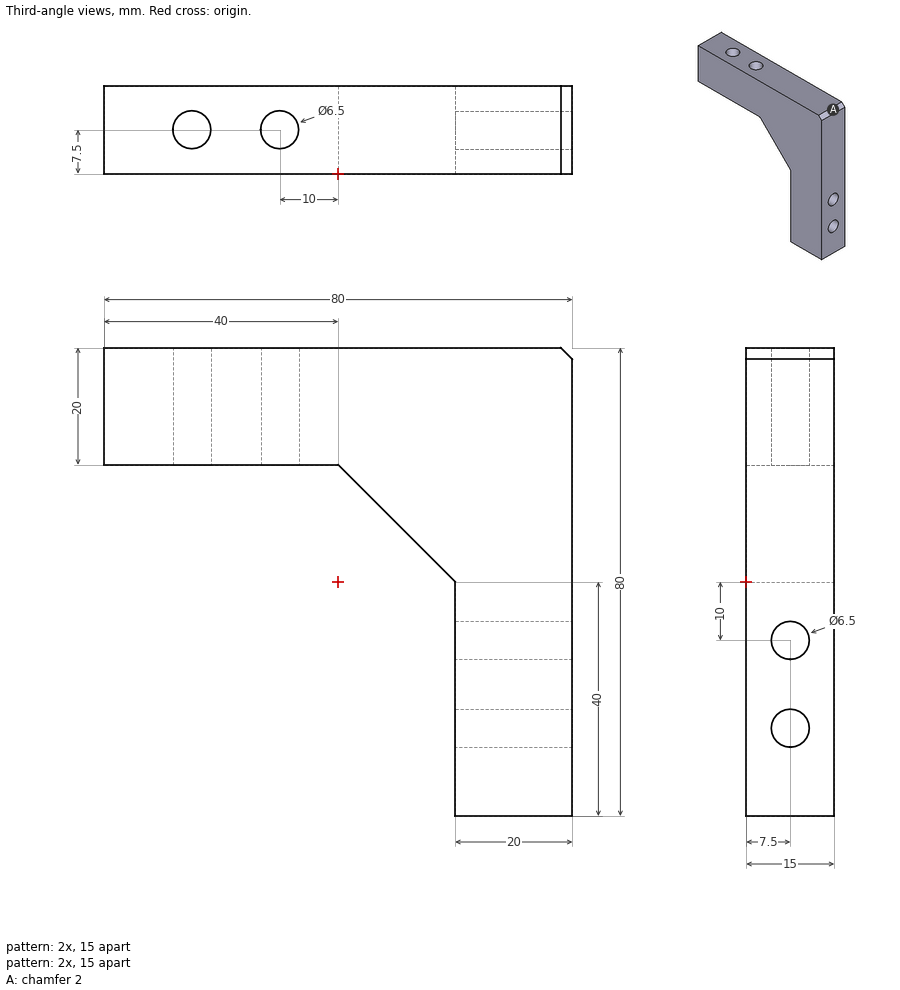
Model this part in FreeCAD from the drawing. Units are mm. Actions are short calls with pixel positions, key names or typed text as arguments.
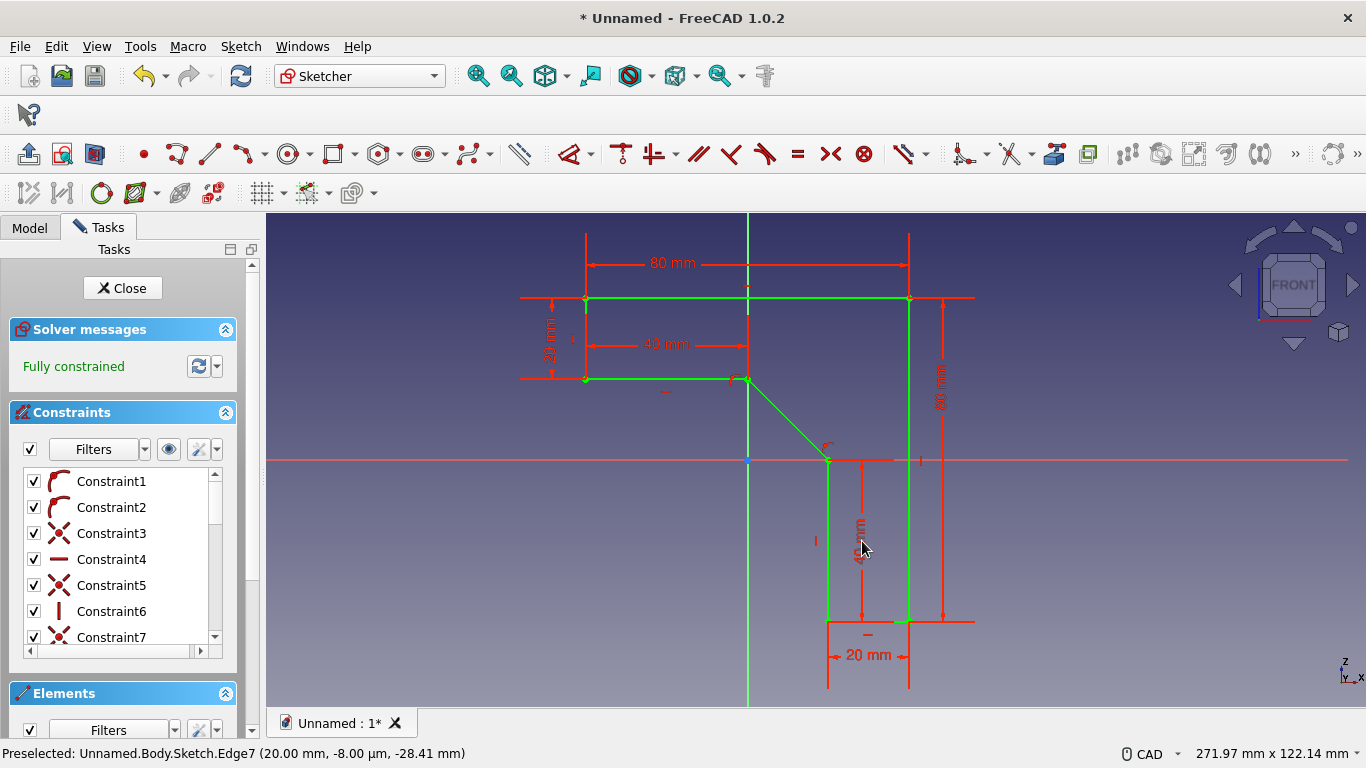
click(123, 288)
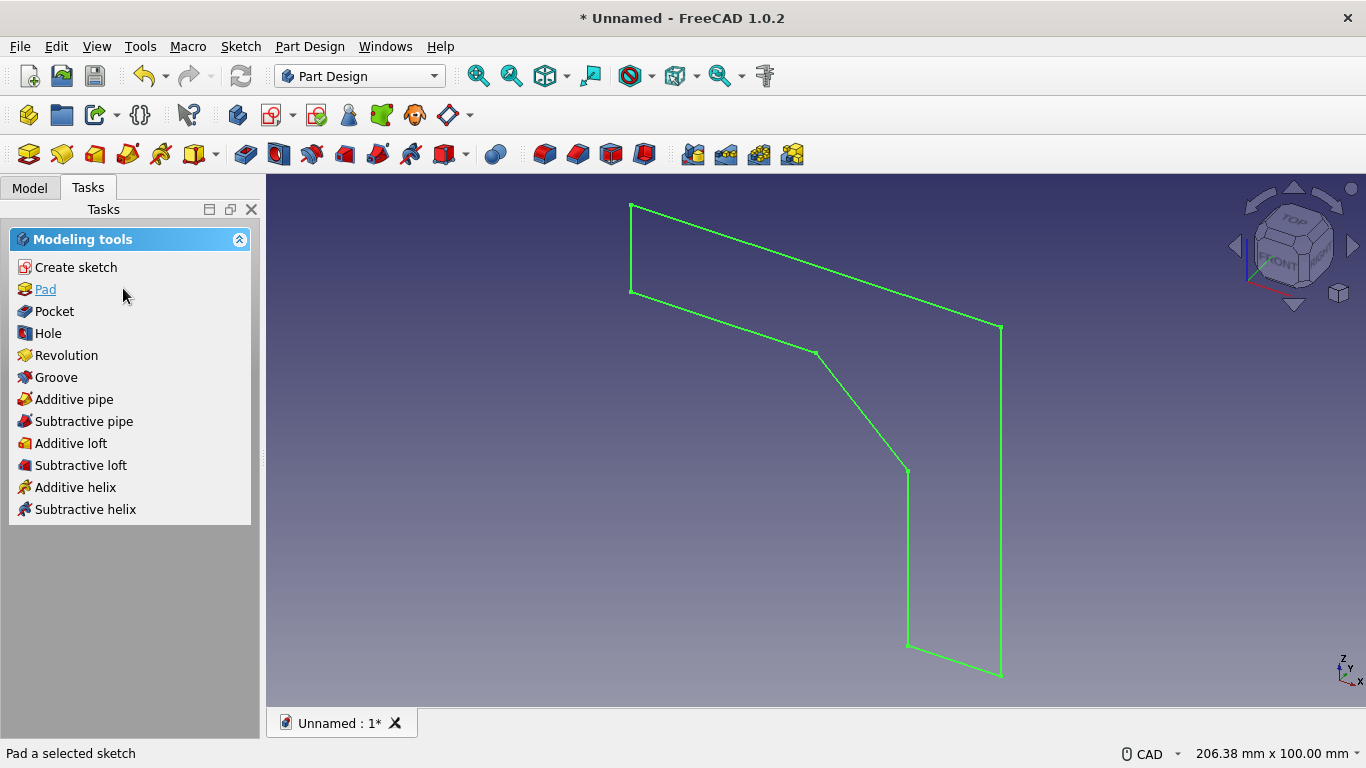
click(29, 154)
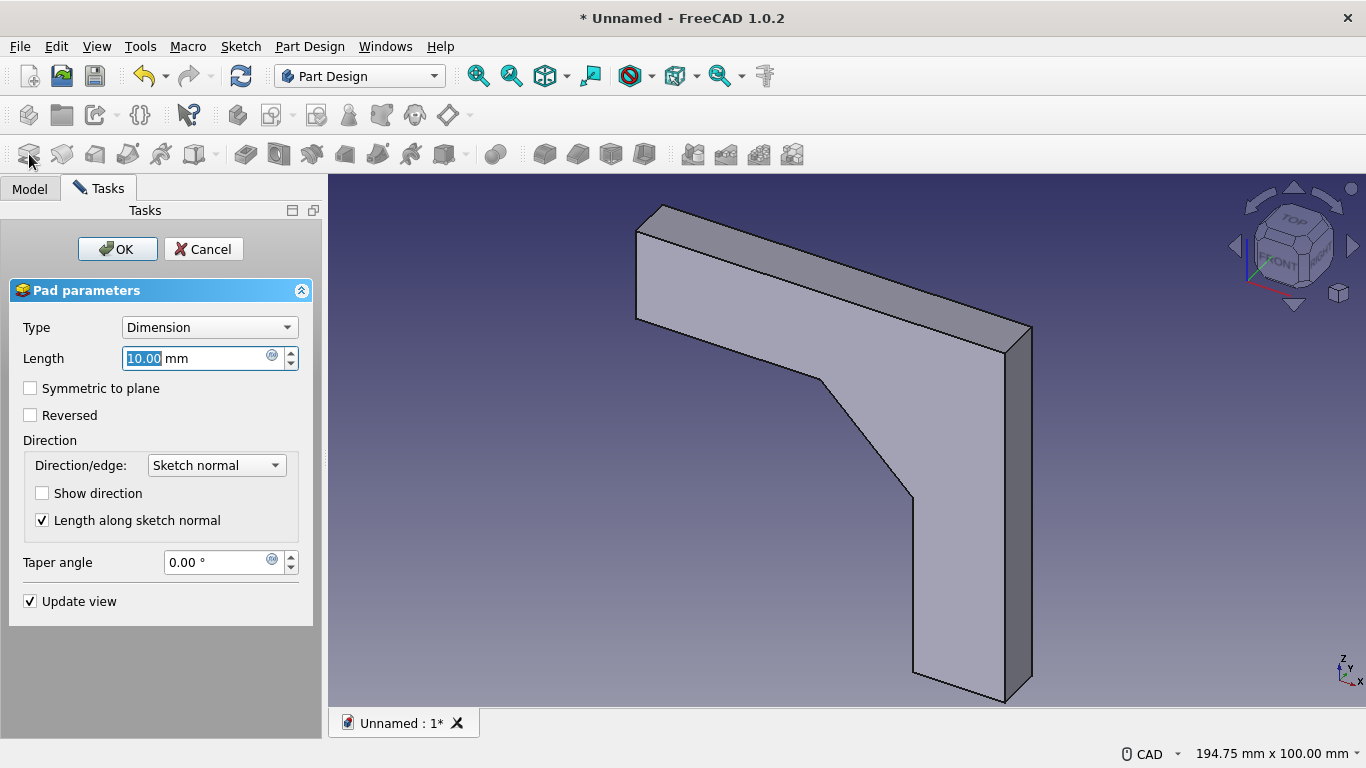
text(15)
key(Tab)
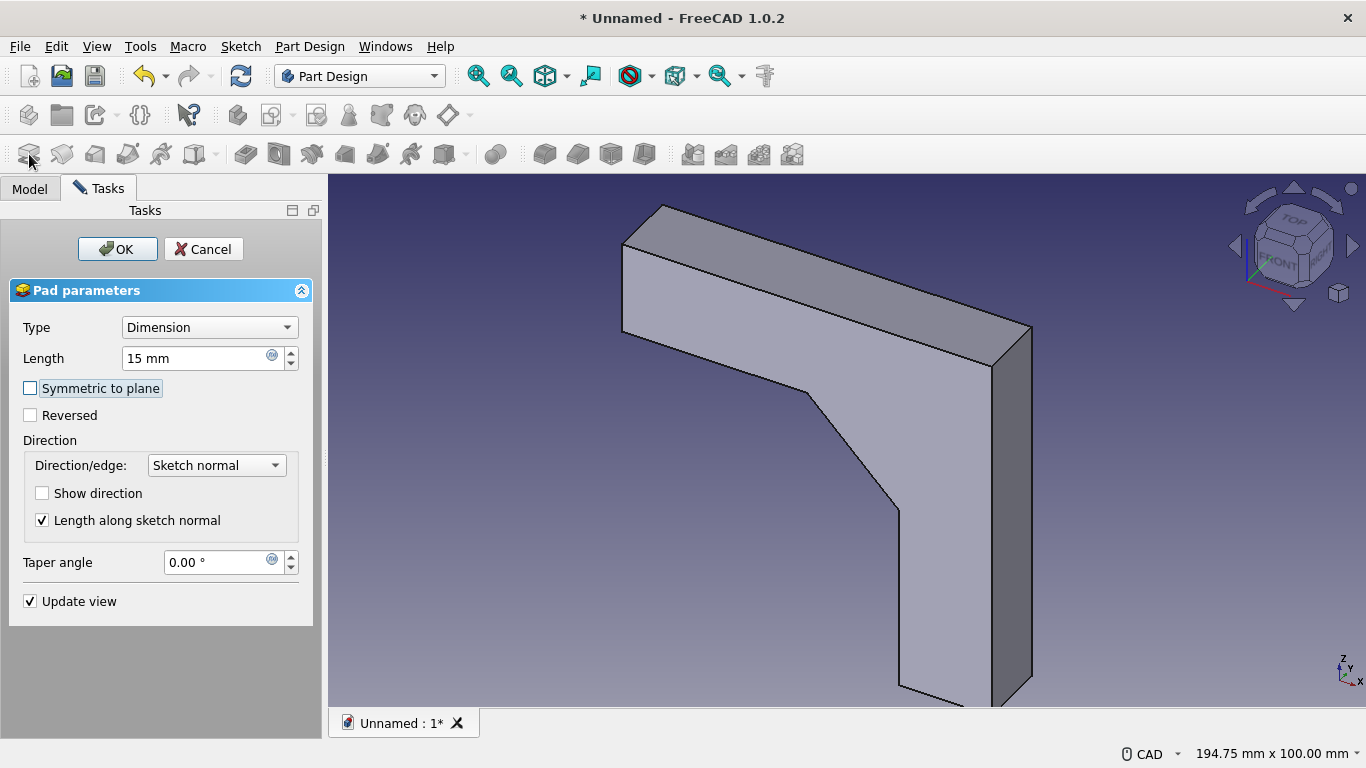
click(31, 415)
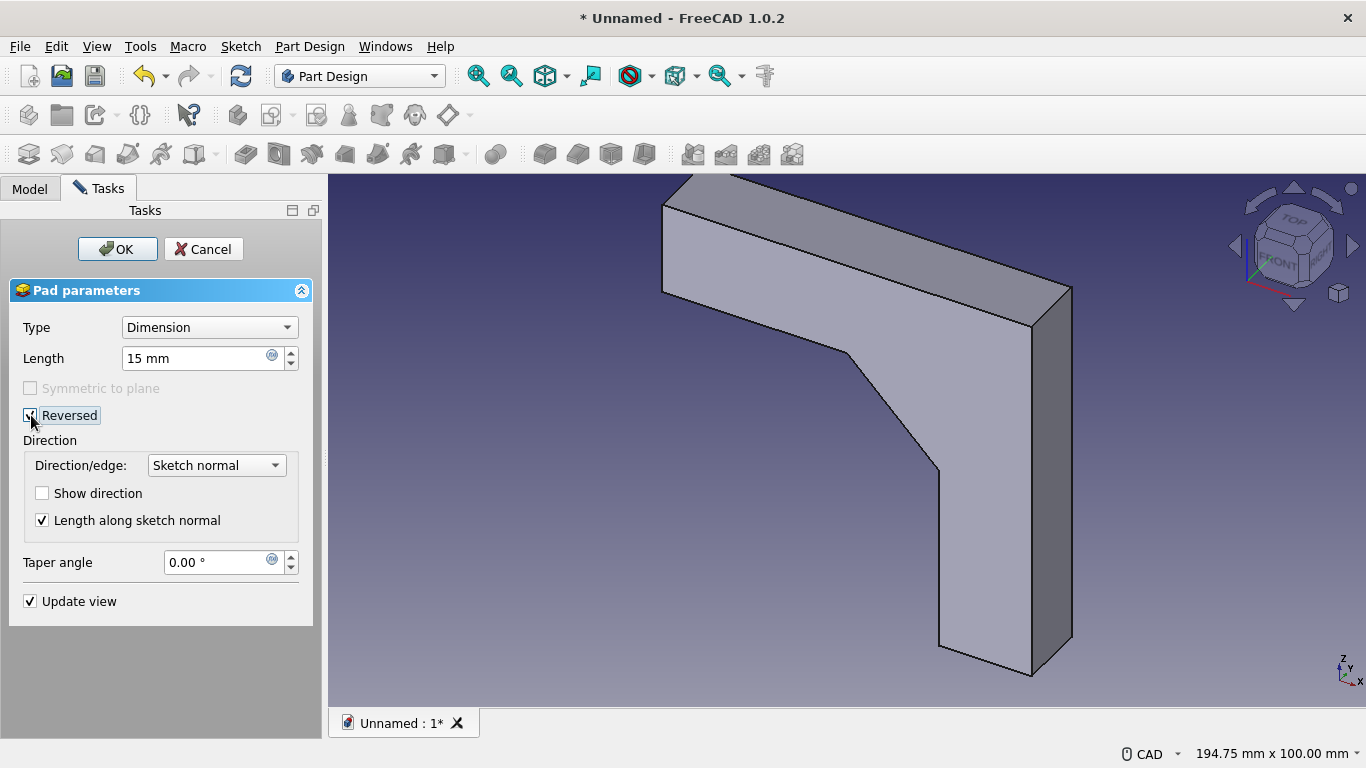
click(118, 249)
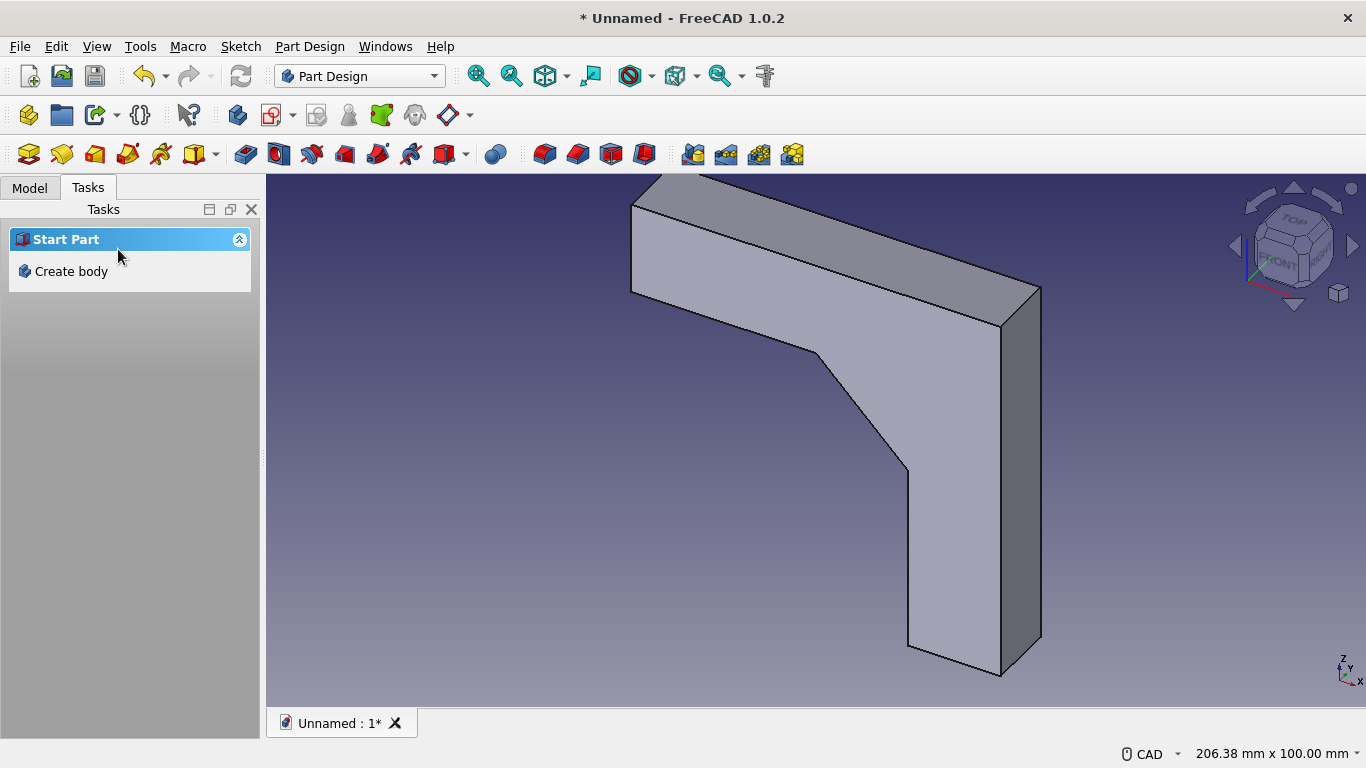
key(v)
key(f)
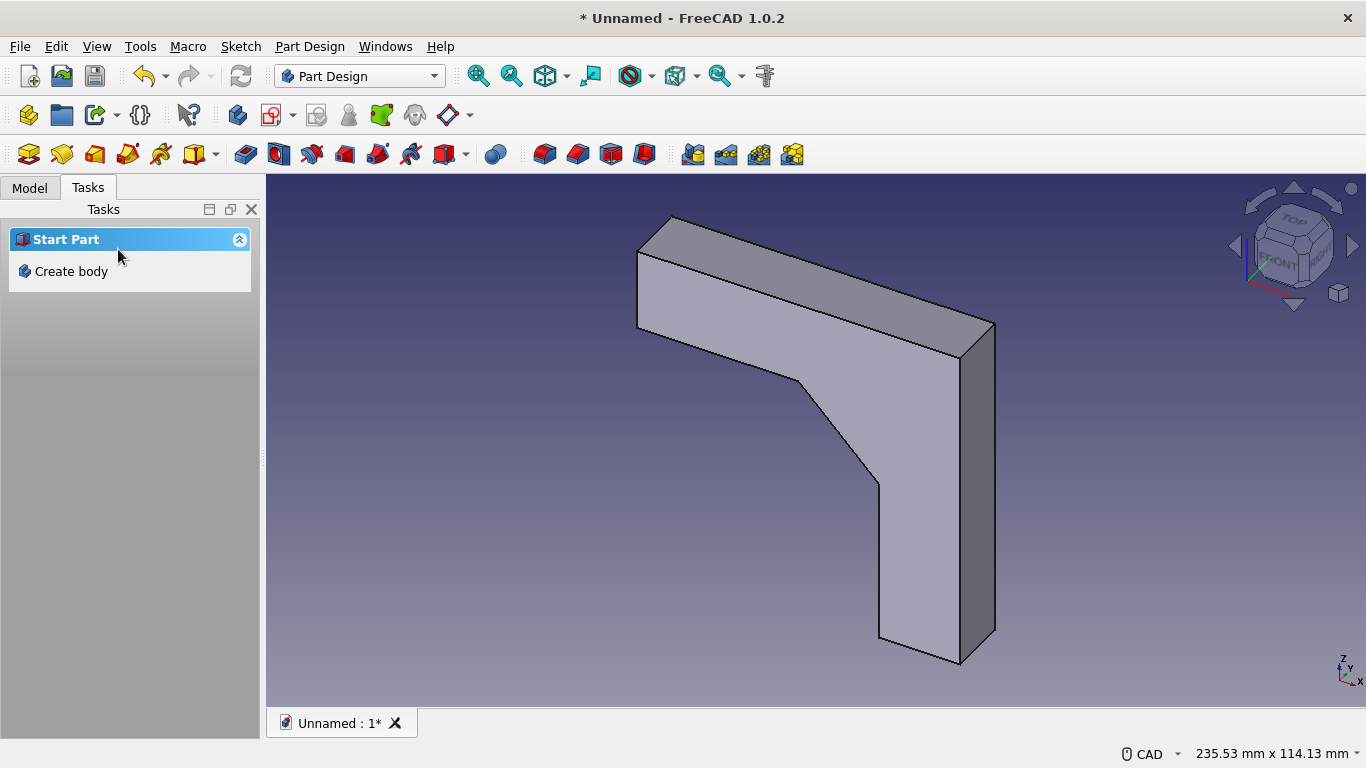
key(5)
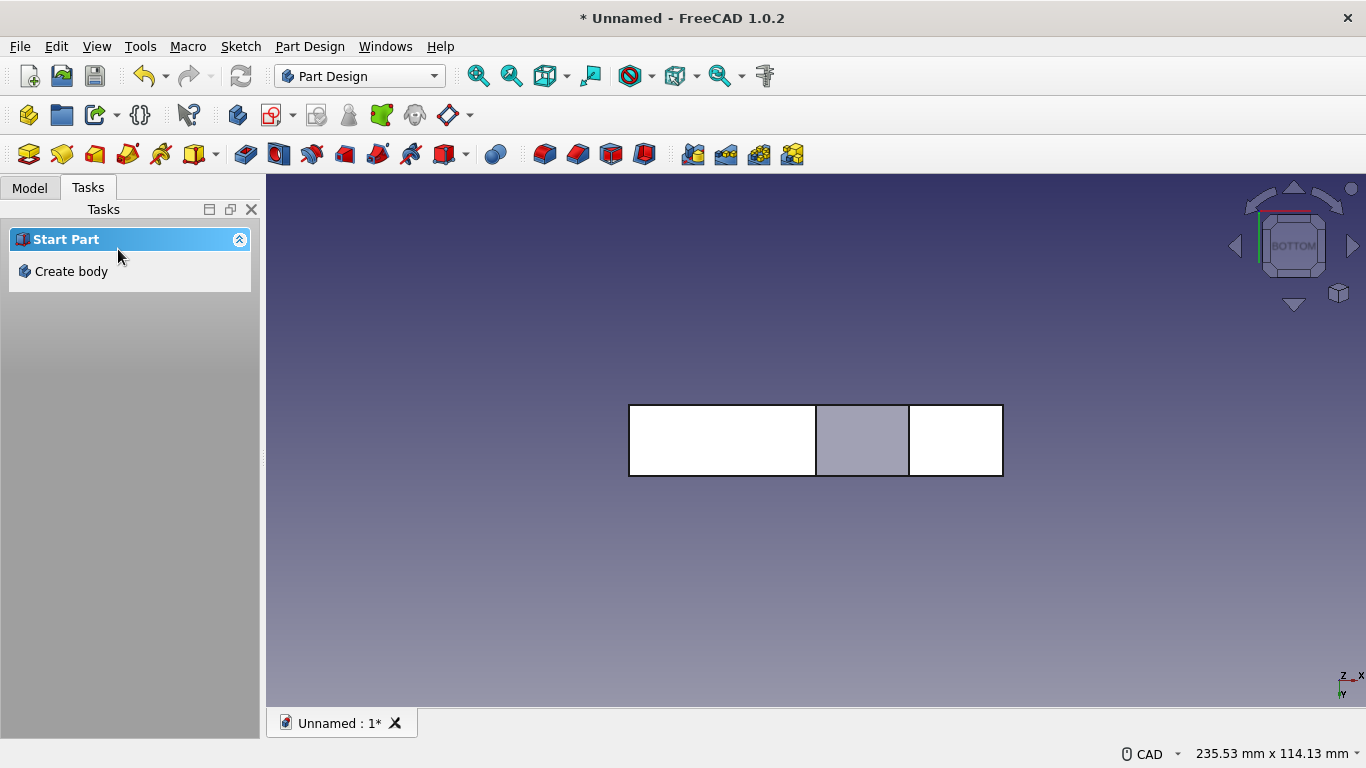
key(v)
key(f)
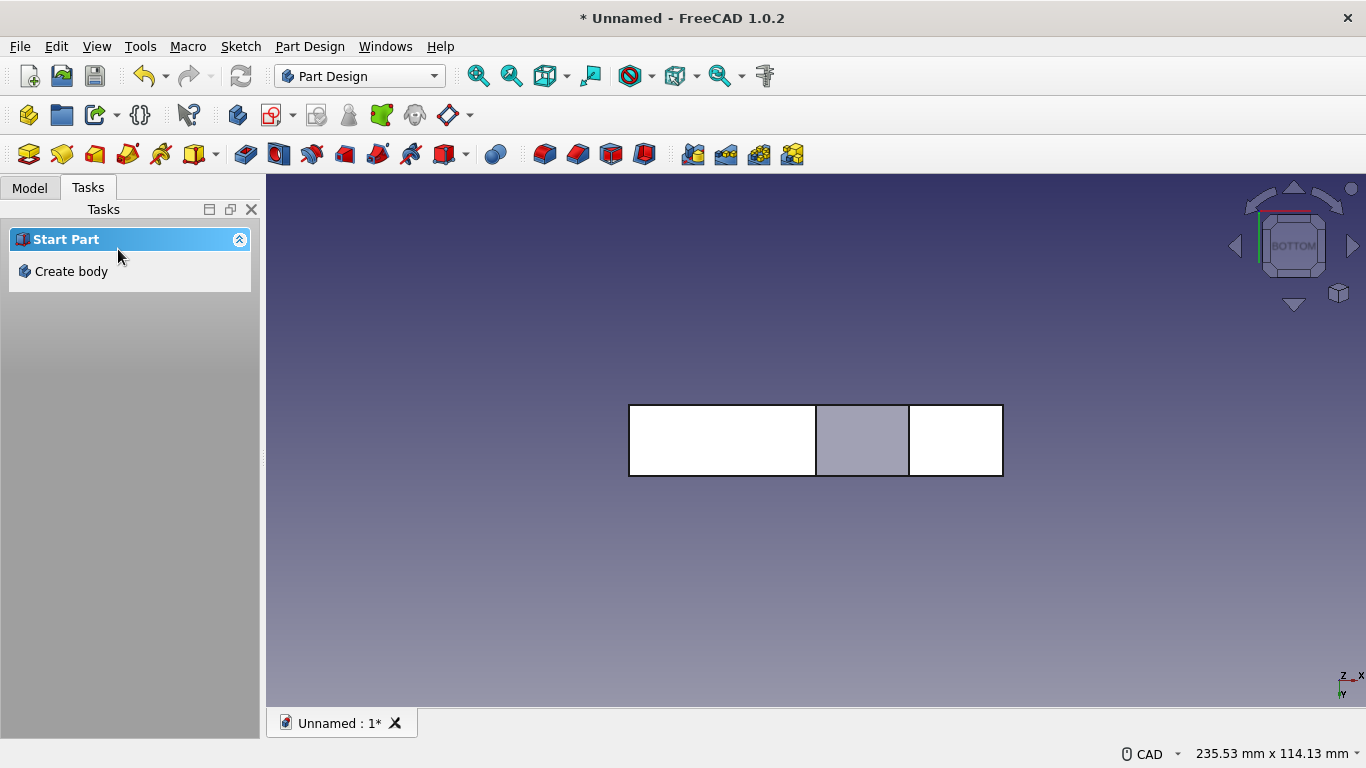
click(776, 439)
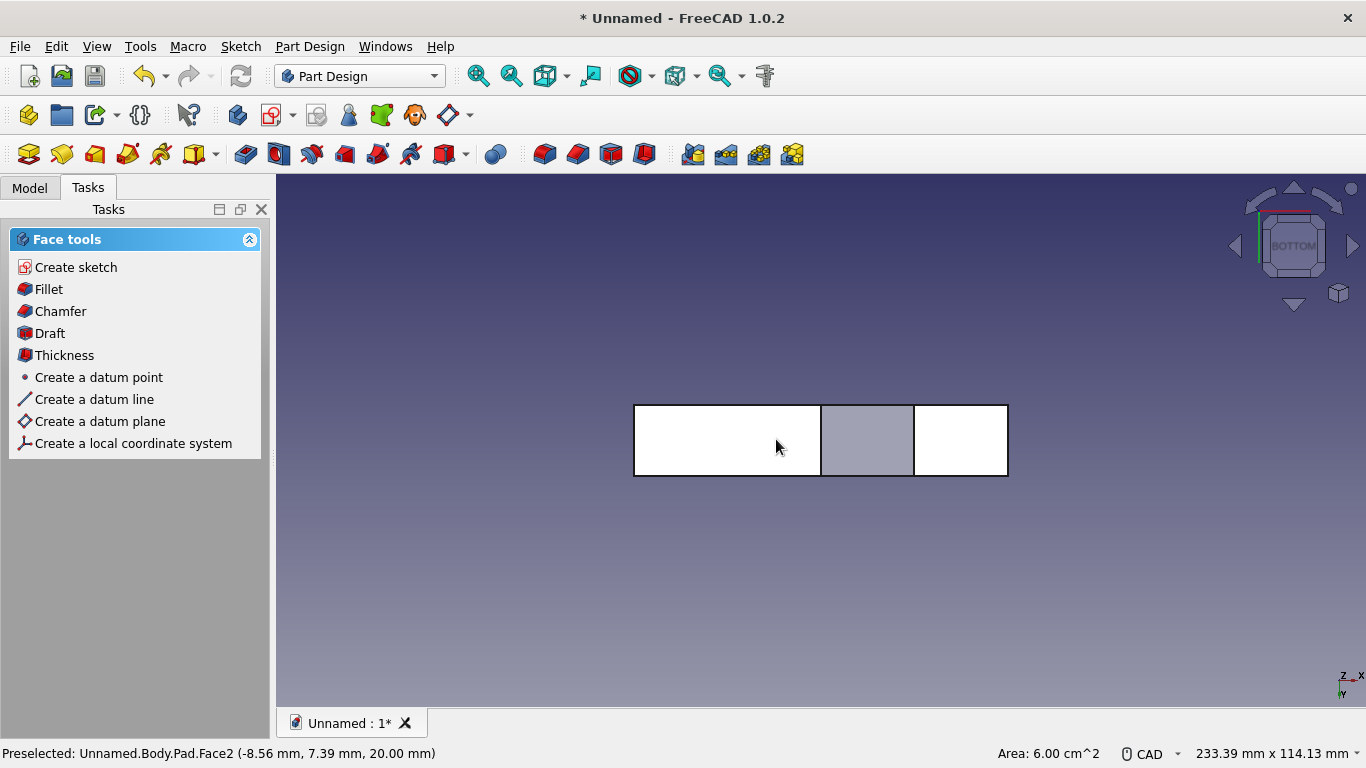
click(270, 116)